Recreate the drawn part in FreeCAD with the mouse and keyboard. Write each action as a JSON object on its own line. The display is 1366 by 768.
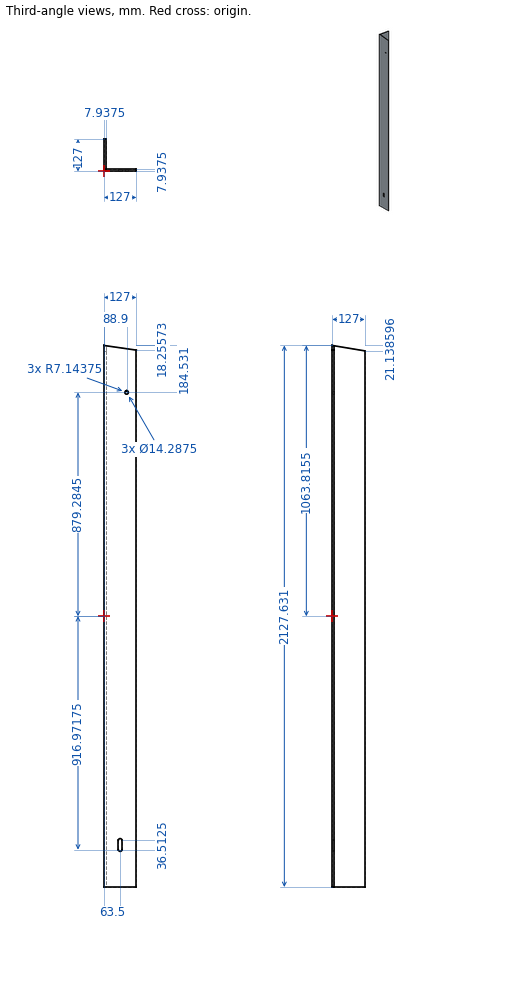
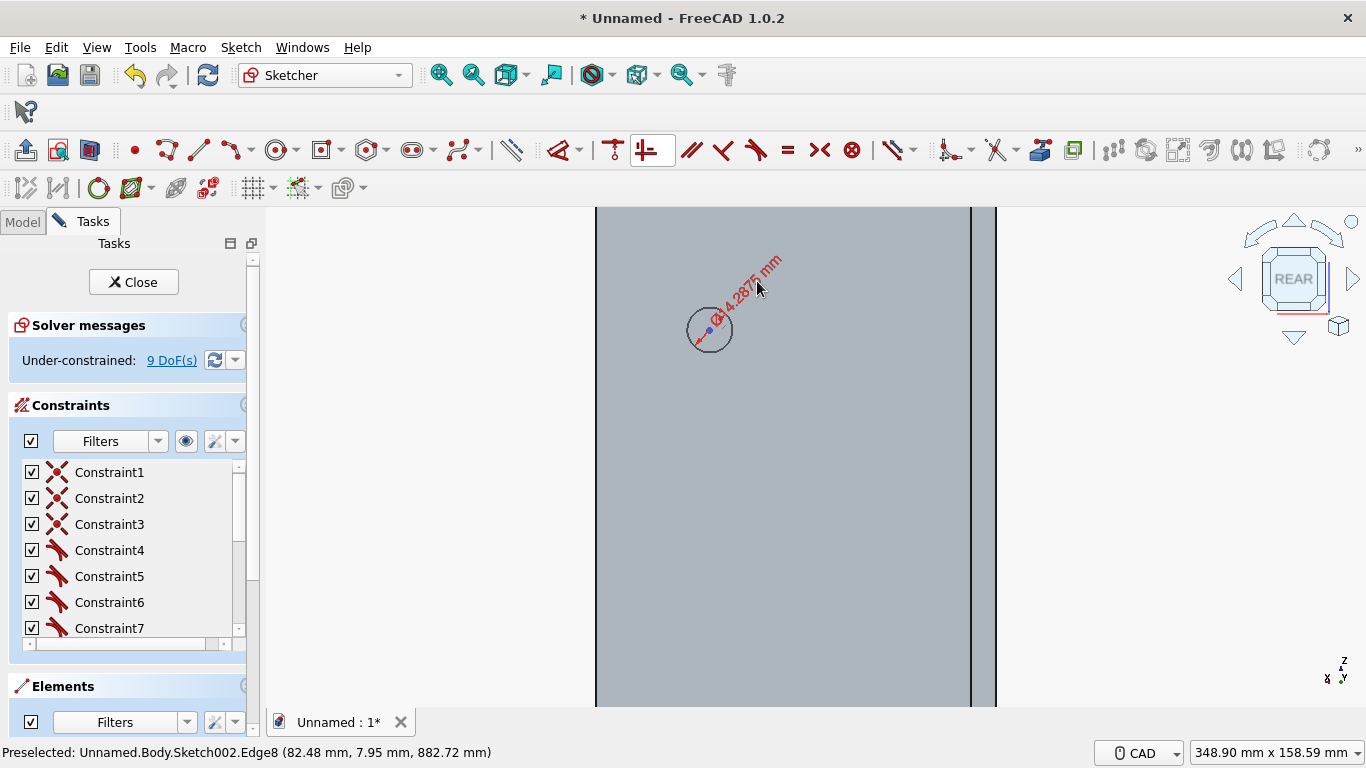
{"action": "scroll", "coordinate": [745, 331], "scroll_direction": "down", "scroll_amount": 15}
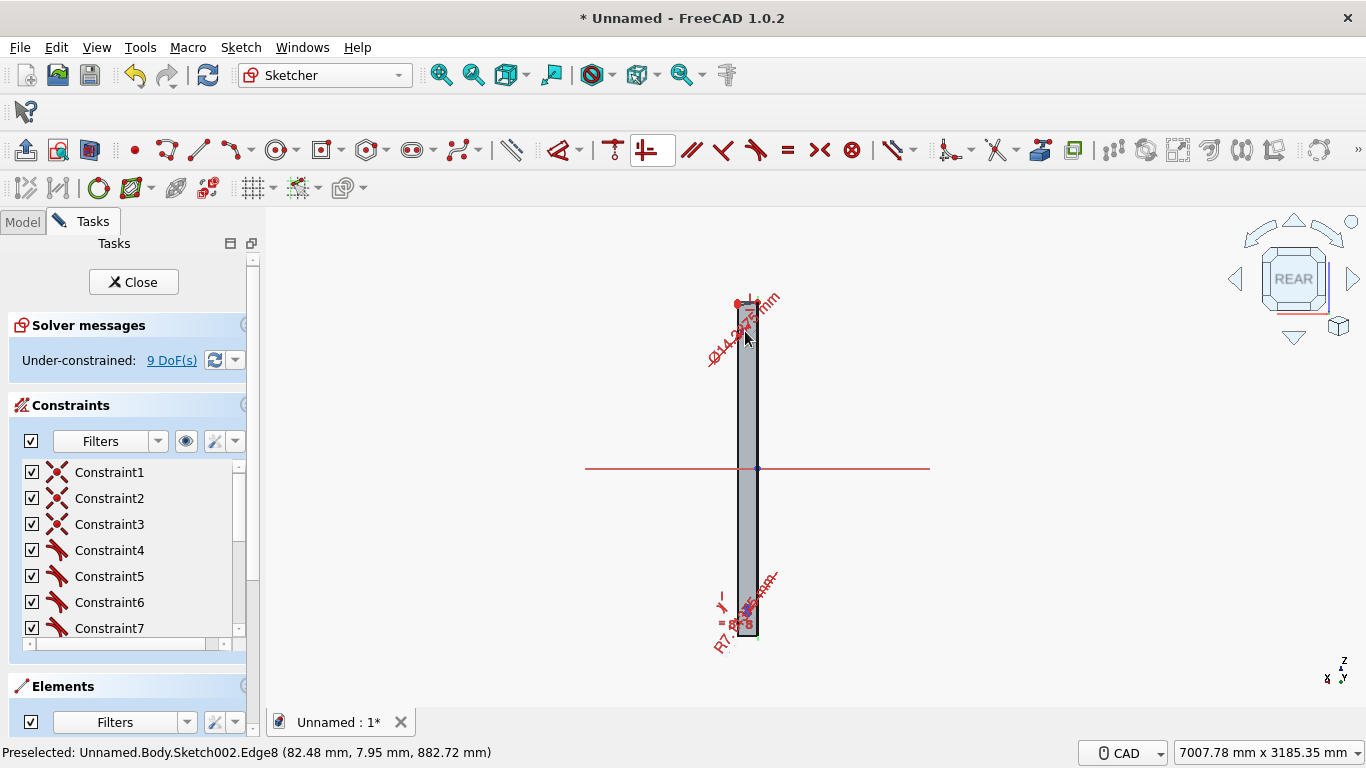
{"action": "left_click", "coordinate": [757, 302]}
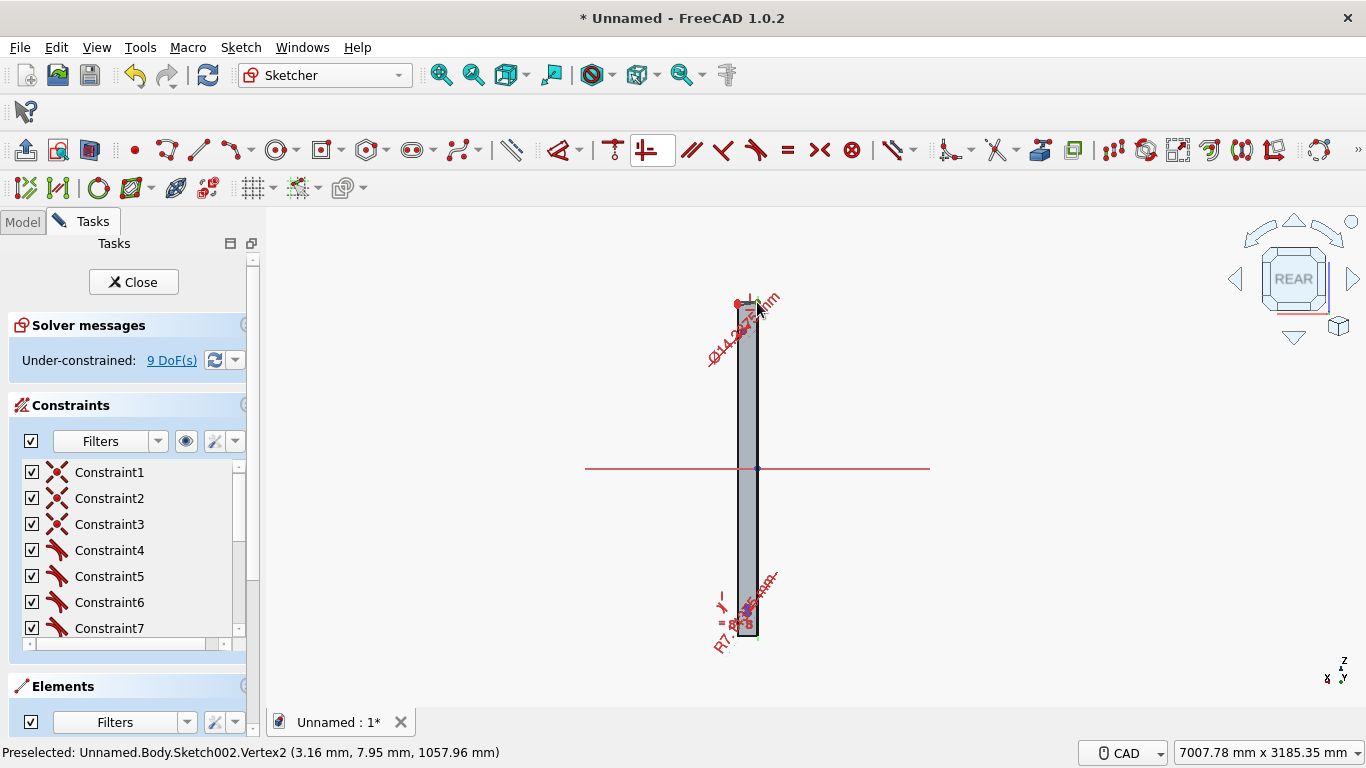
{"action": "left_click", "coordinate": [758, 552]}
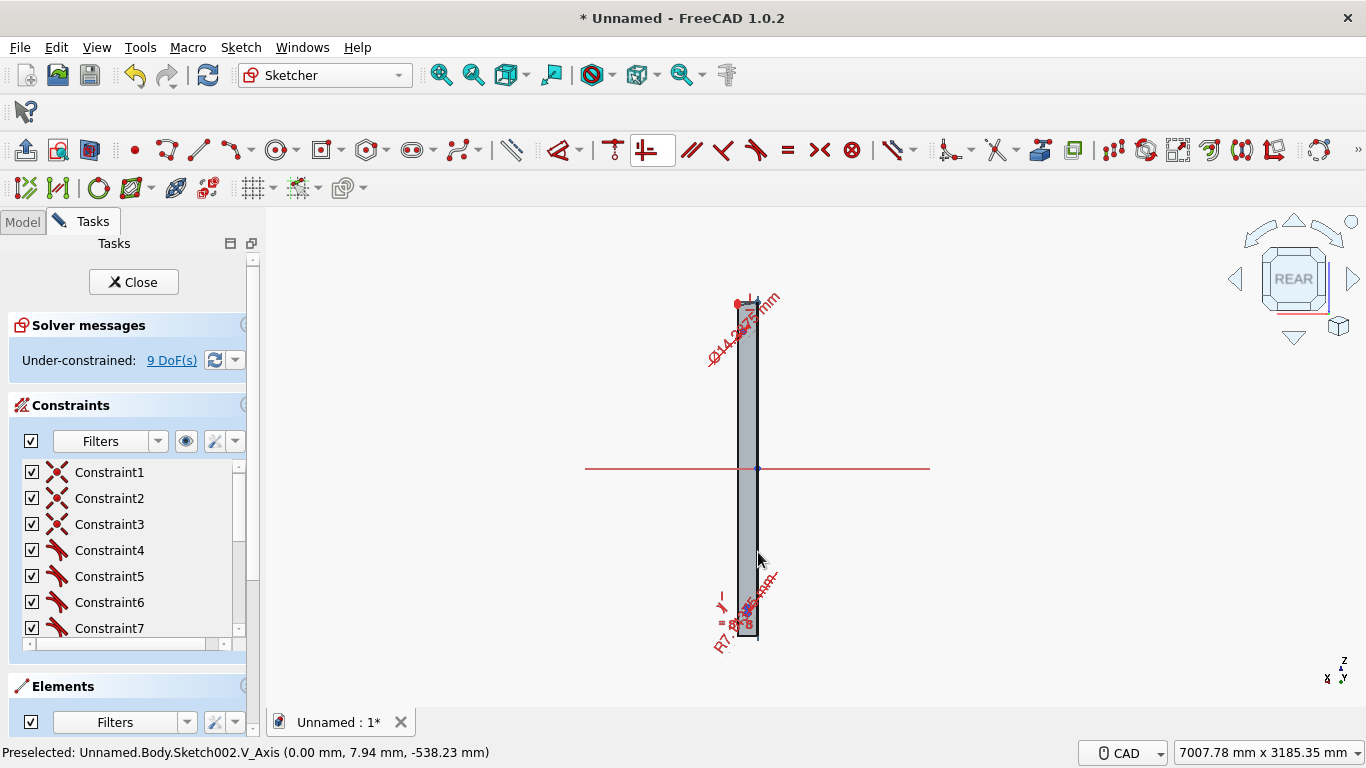
{"action": "left_click", "coordinate": [614, 150]}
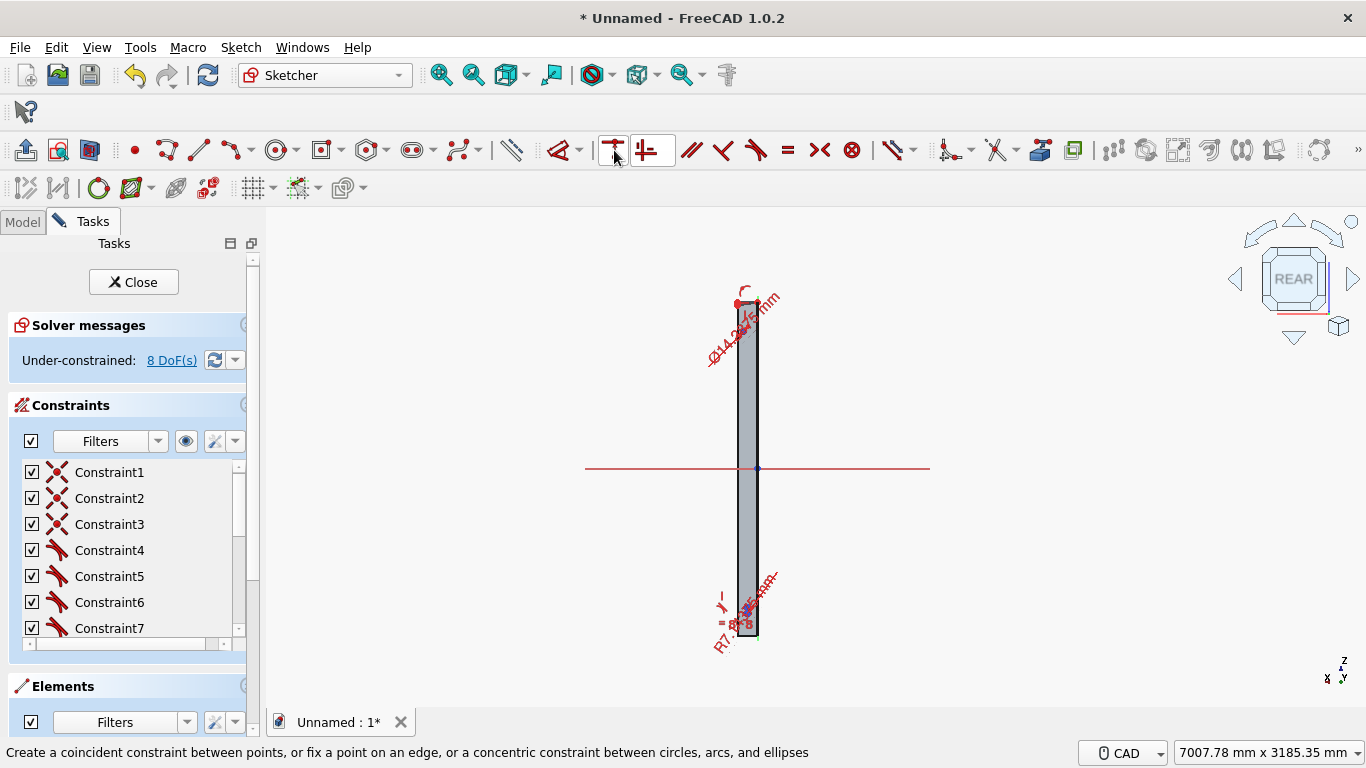
{"action": "key", "text": "d"}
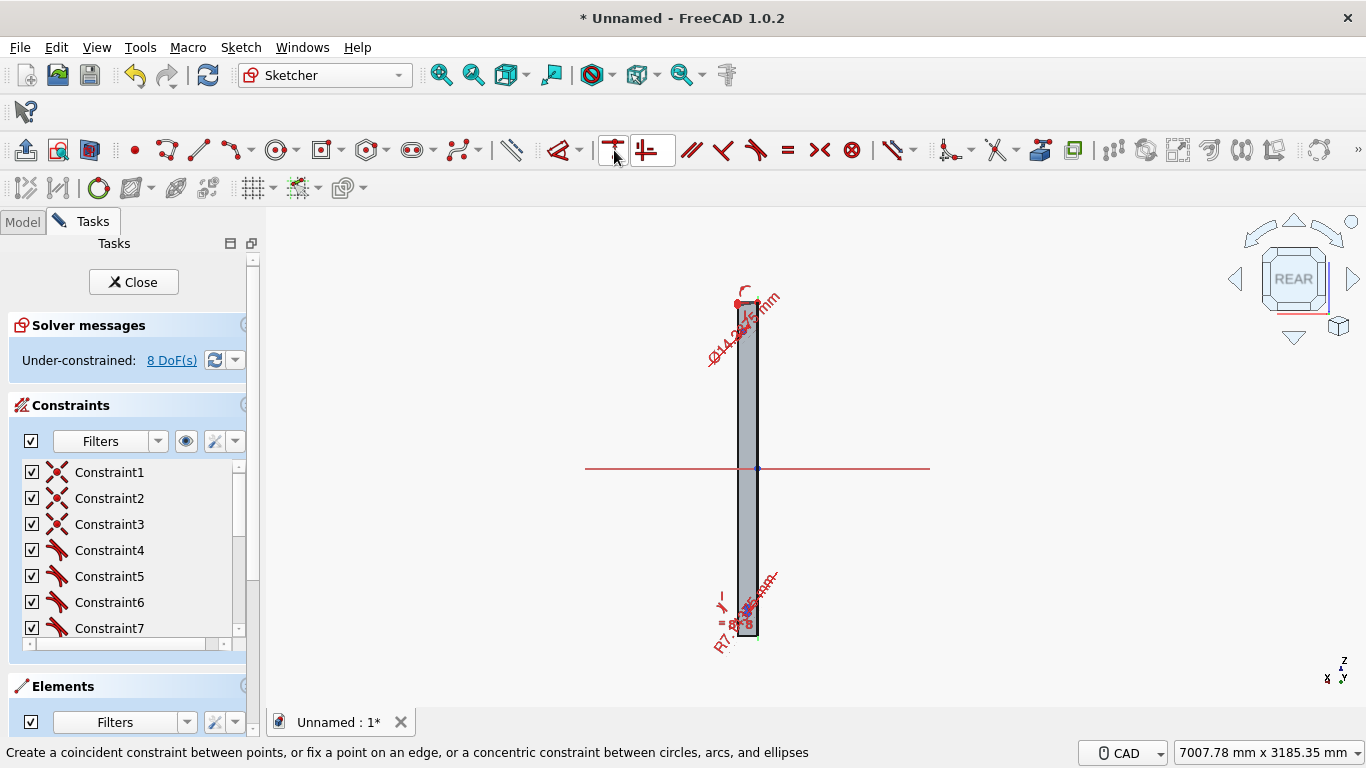
{"action": "scroll", "coordinate": [742, 302], "scroll_direction": "up", "scroll_amount": 9}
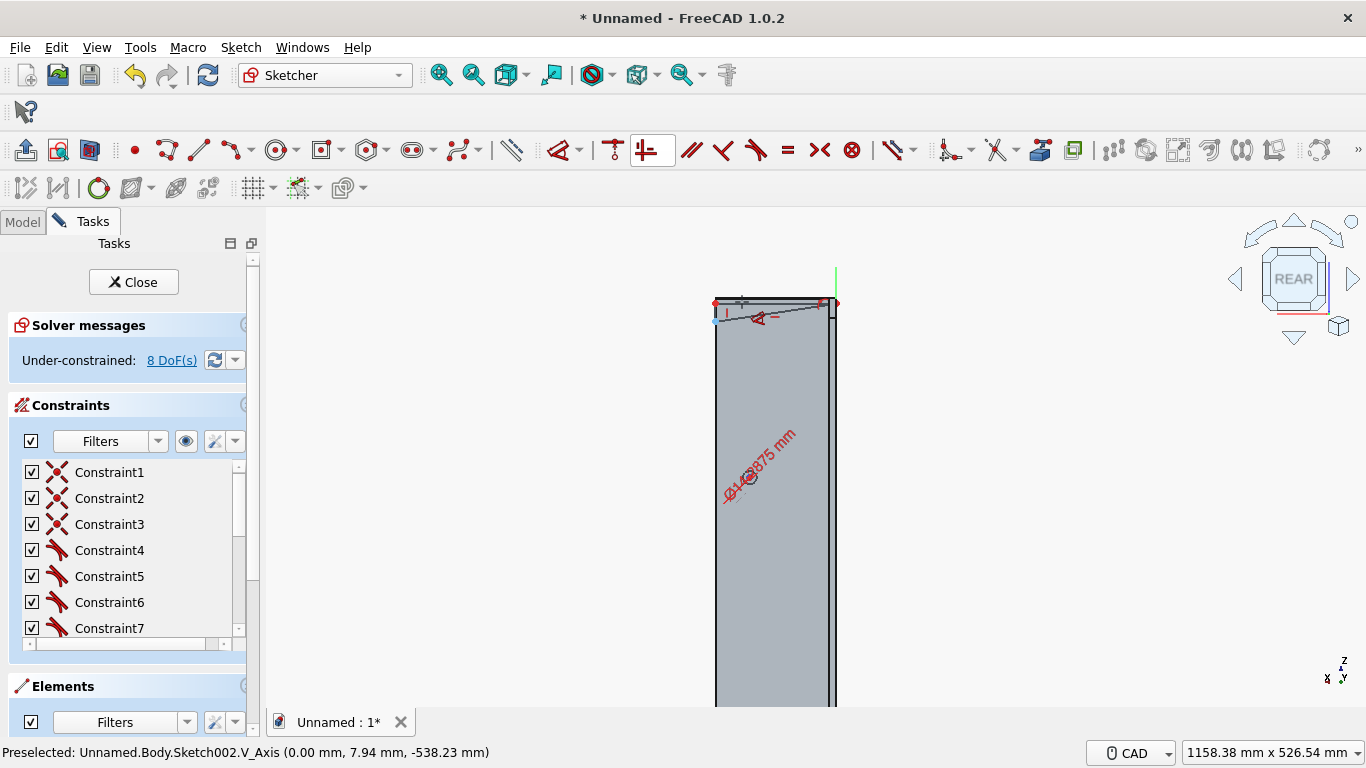
{"action": "left_click", "coordinate": [740, 304]}
{"action": "left_click", "coordinate": [776, 270]}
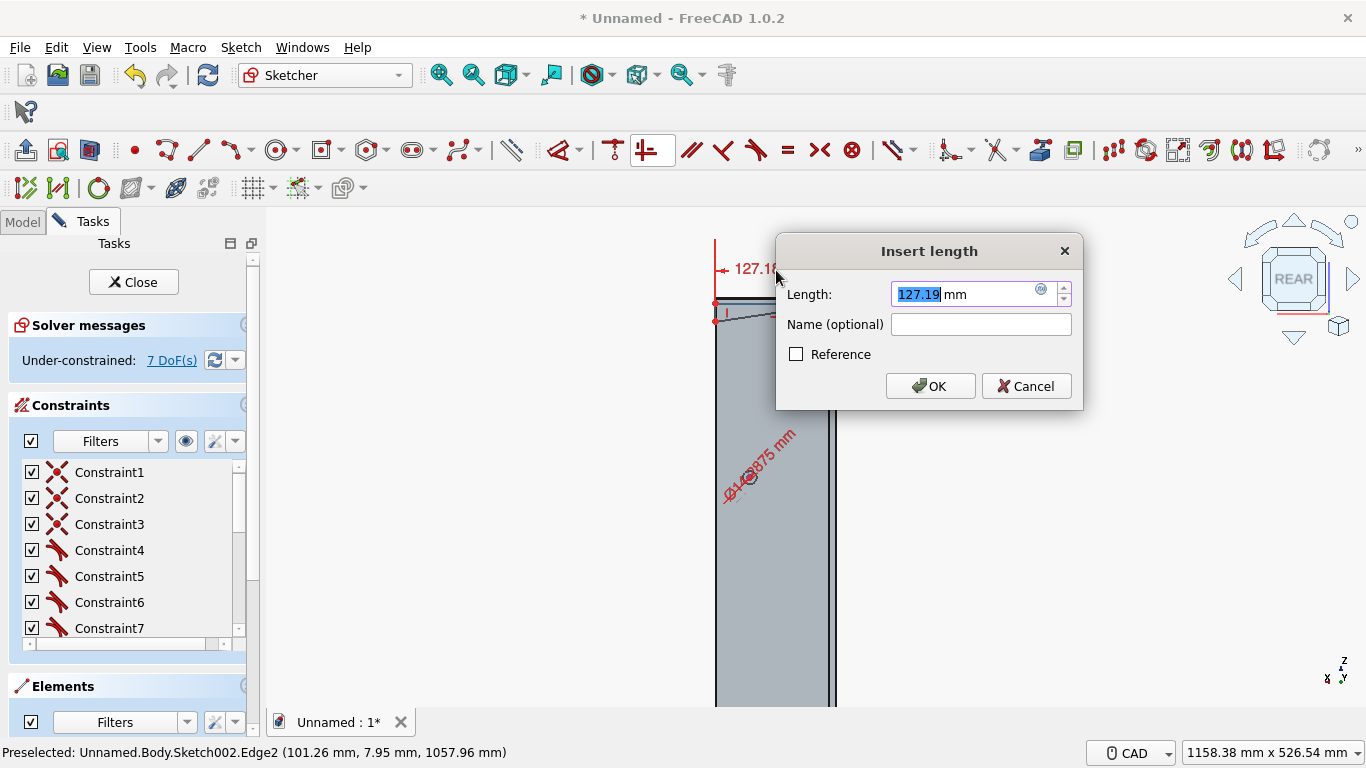
{"action": "type", "text": "127"}
{"action": "key", "text": "Return"}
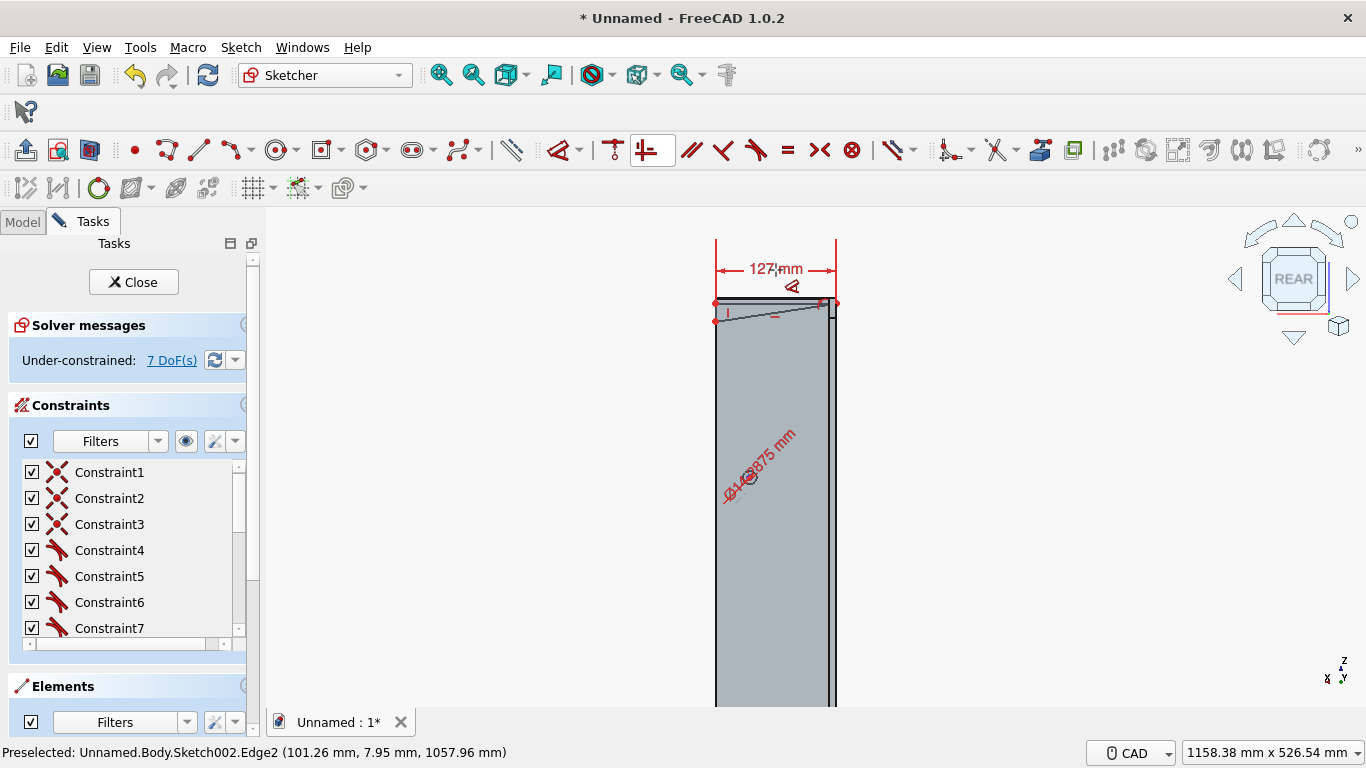
{"action": "left_click", "coordinate": [750, 478]}
{"action": "left_click", "coordinate": [793, 420]}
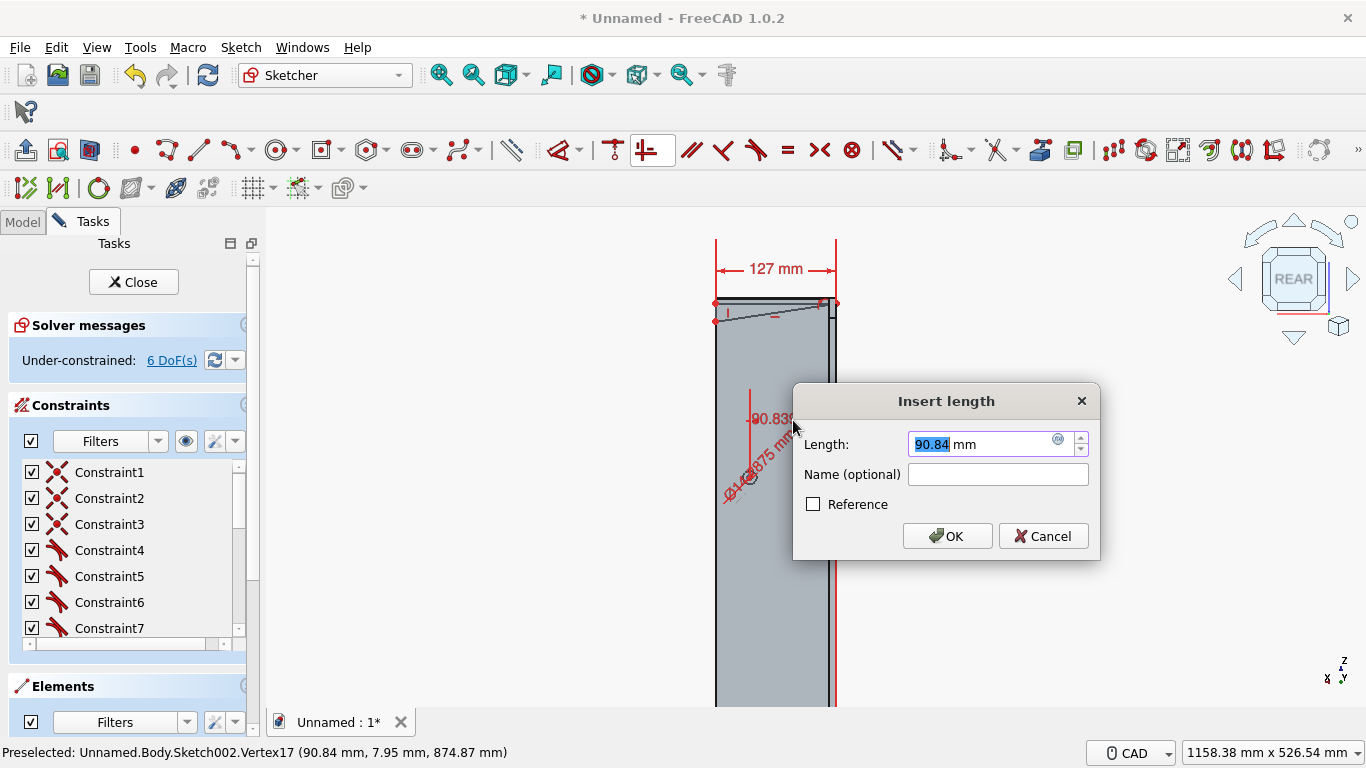
{"action": "type", "text": "88.9"}
{"action": "key", "text": "Return"}